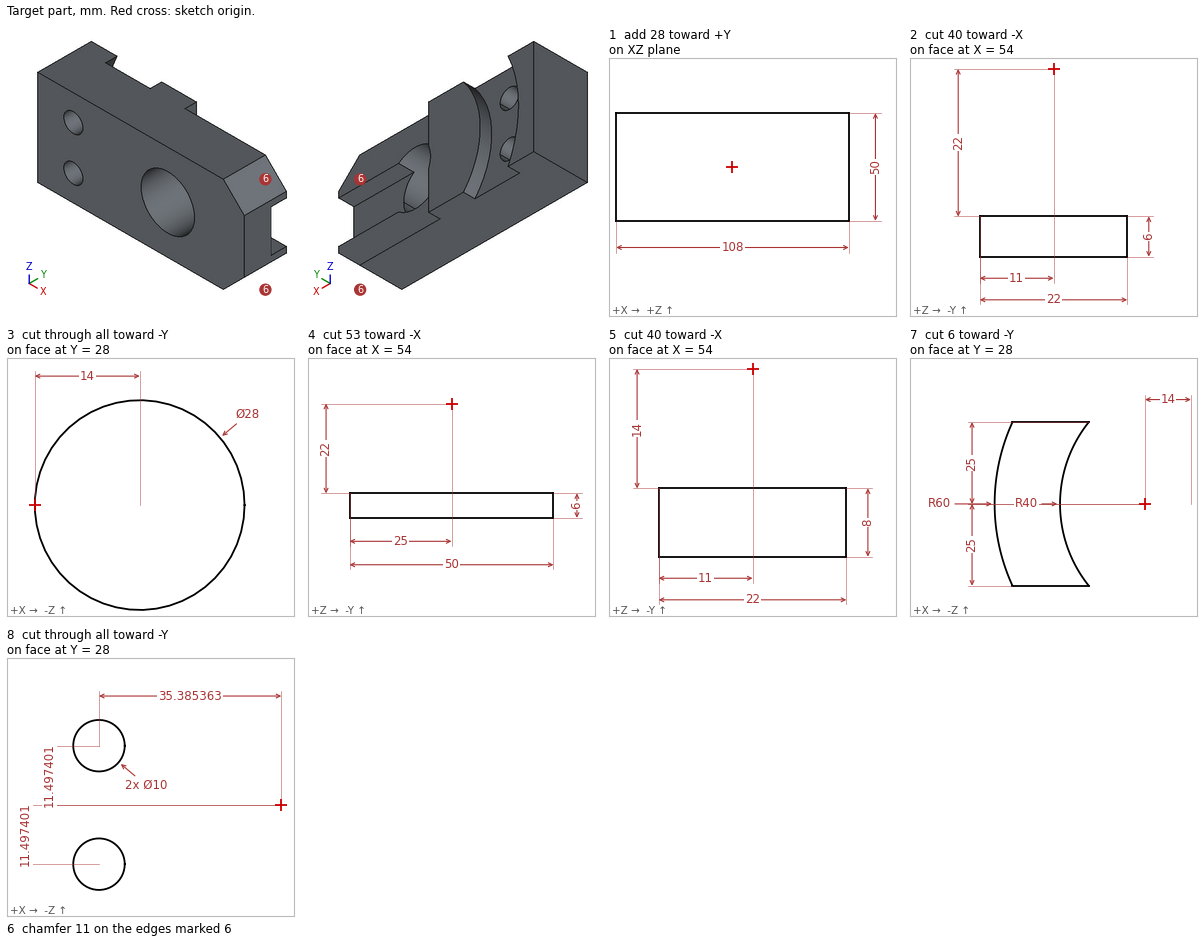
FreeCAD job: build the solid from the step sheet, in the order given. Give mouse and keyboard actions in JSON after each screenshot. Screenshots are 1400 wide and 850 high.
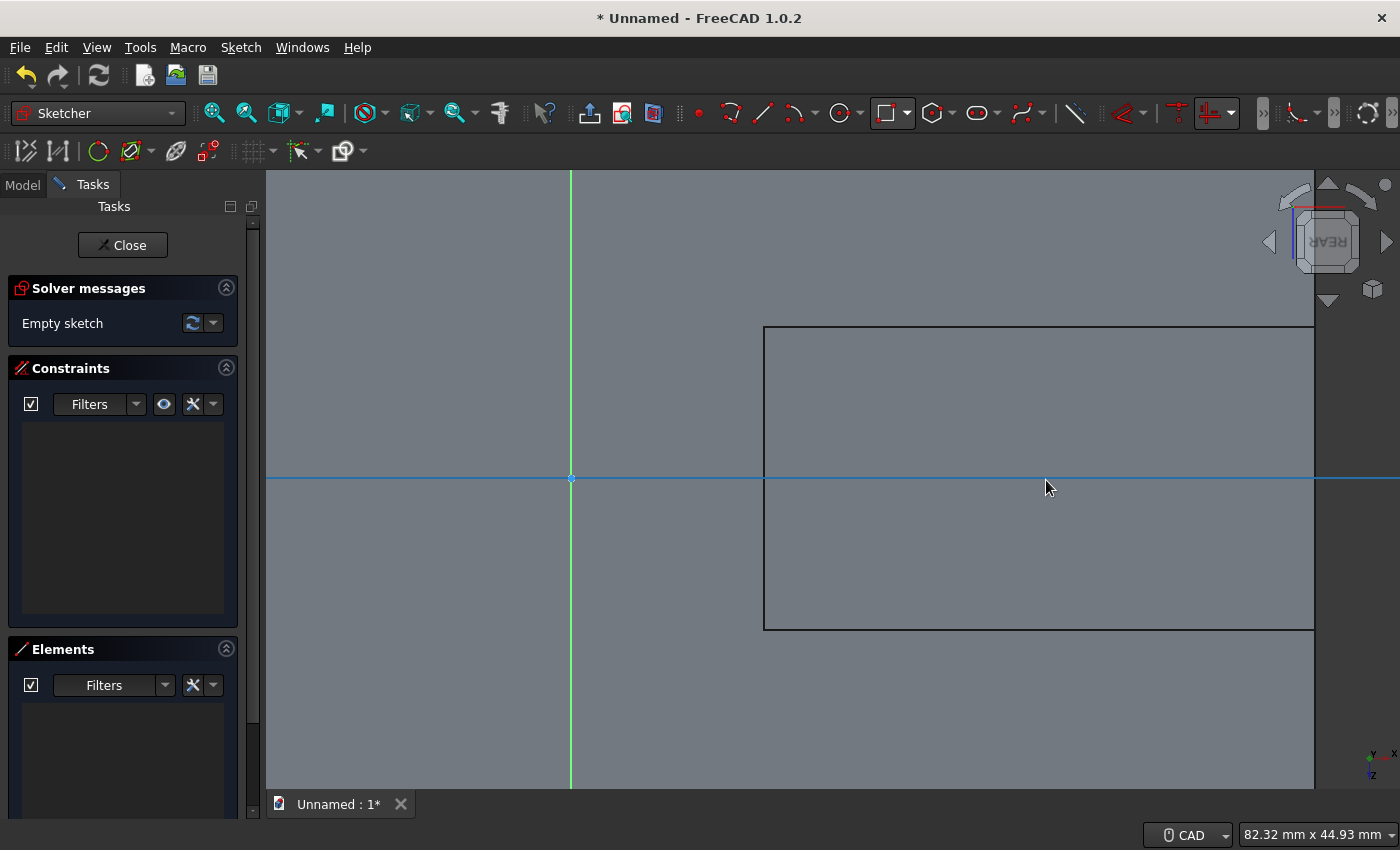
{"action": "key", "text": "g c"}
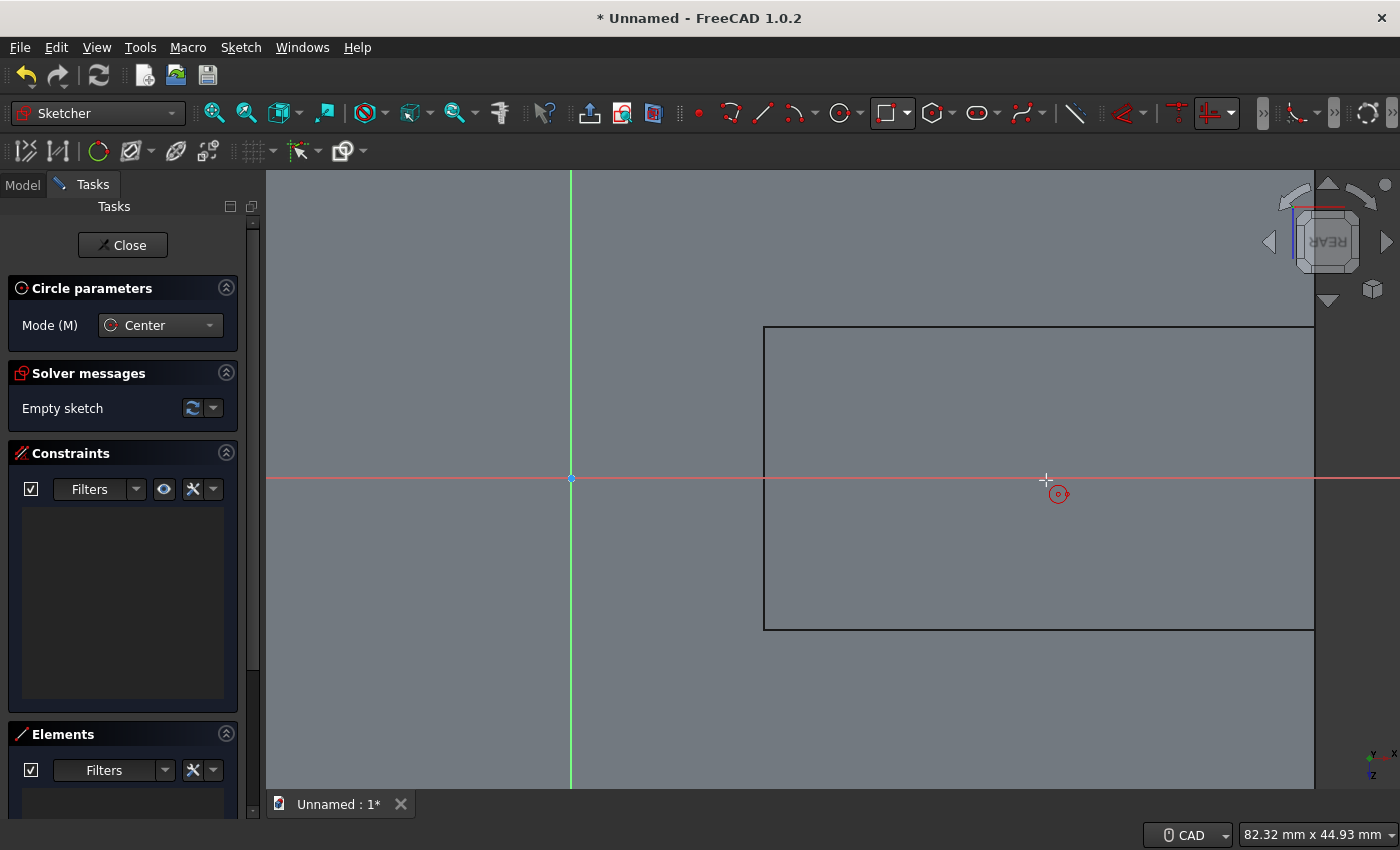
{"action": "left_click", "coordinate": [764, 478]}
{"action": "mouse_move", "coordinate": [900, 342]}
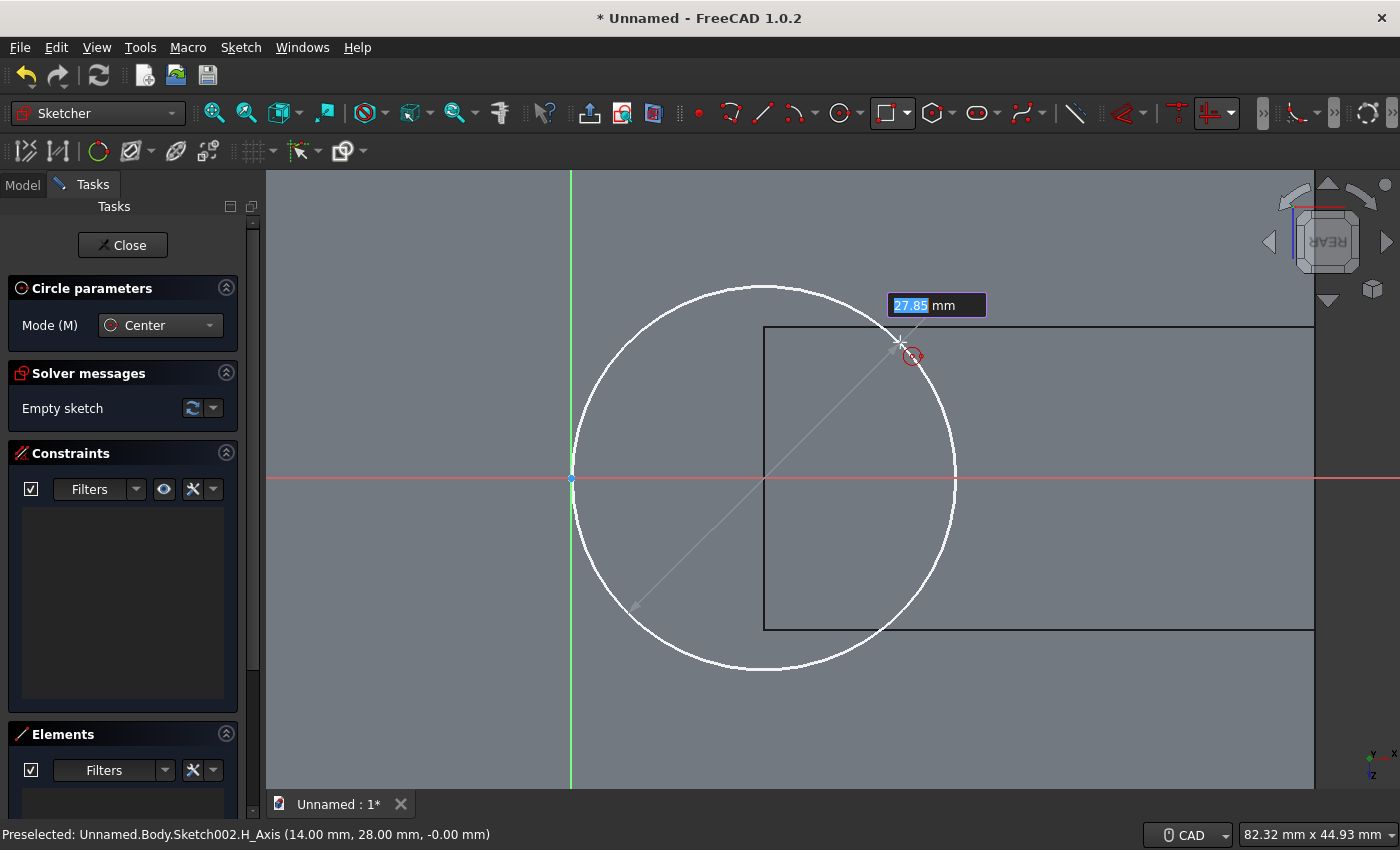
{"action": "type", "text": "28"}
{"action": "key", "text": "Return"}
{"action": "key", "text": "Escape"}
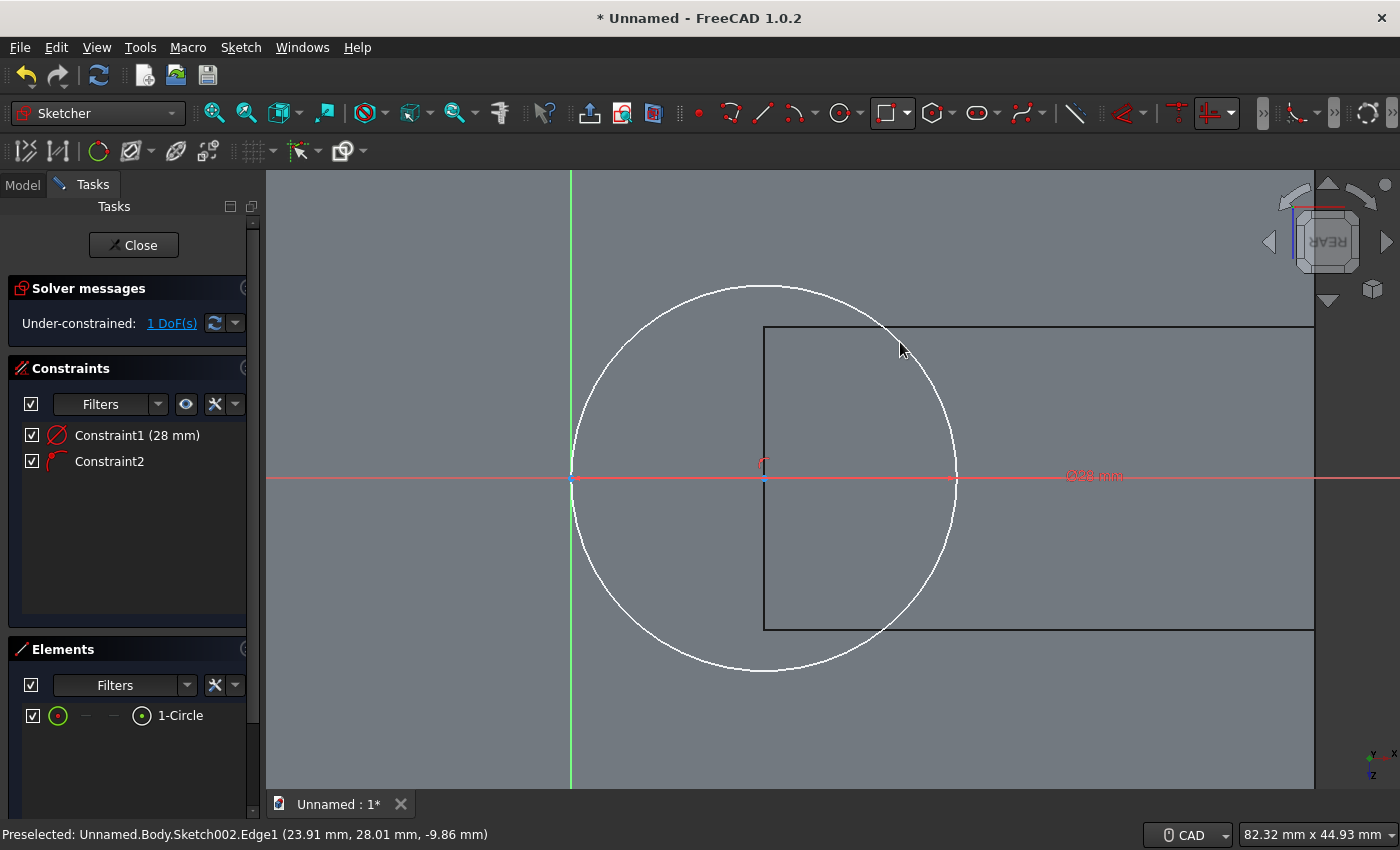
{"action": "key", "text": "d"}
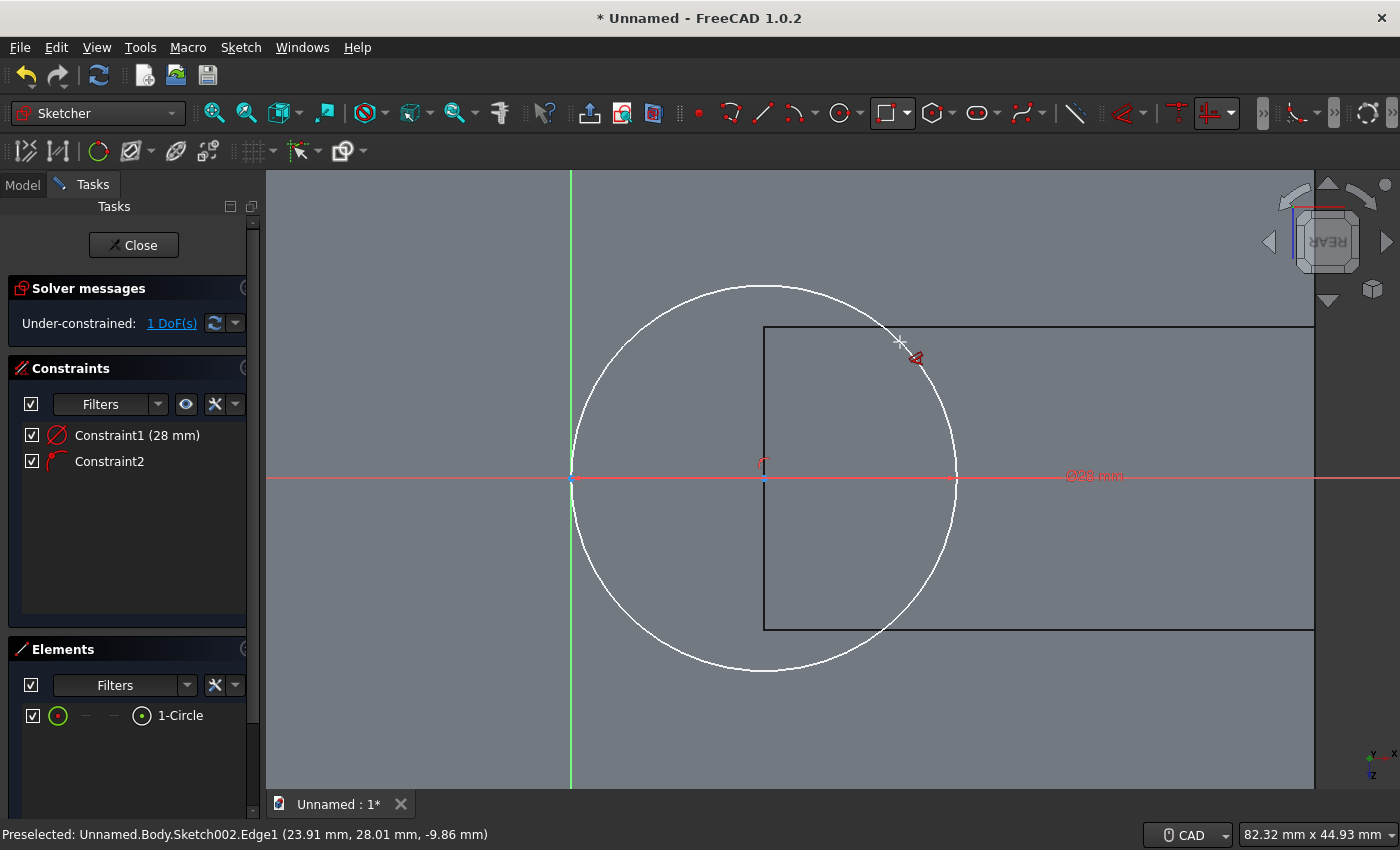
{"action": "left_click", "coordinate": [764, 478]}
{"action": "left_click", "coordinate": [668, 512]}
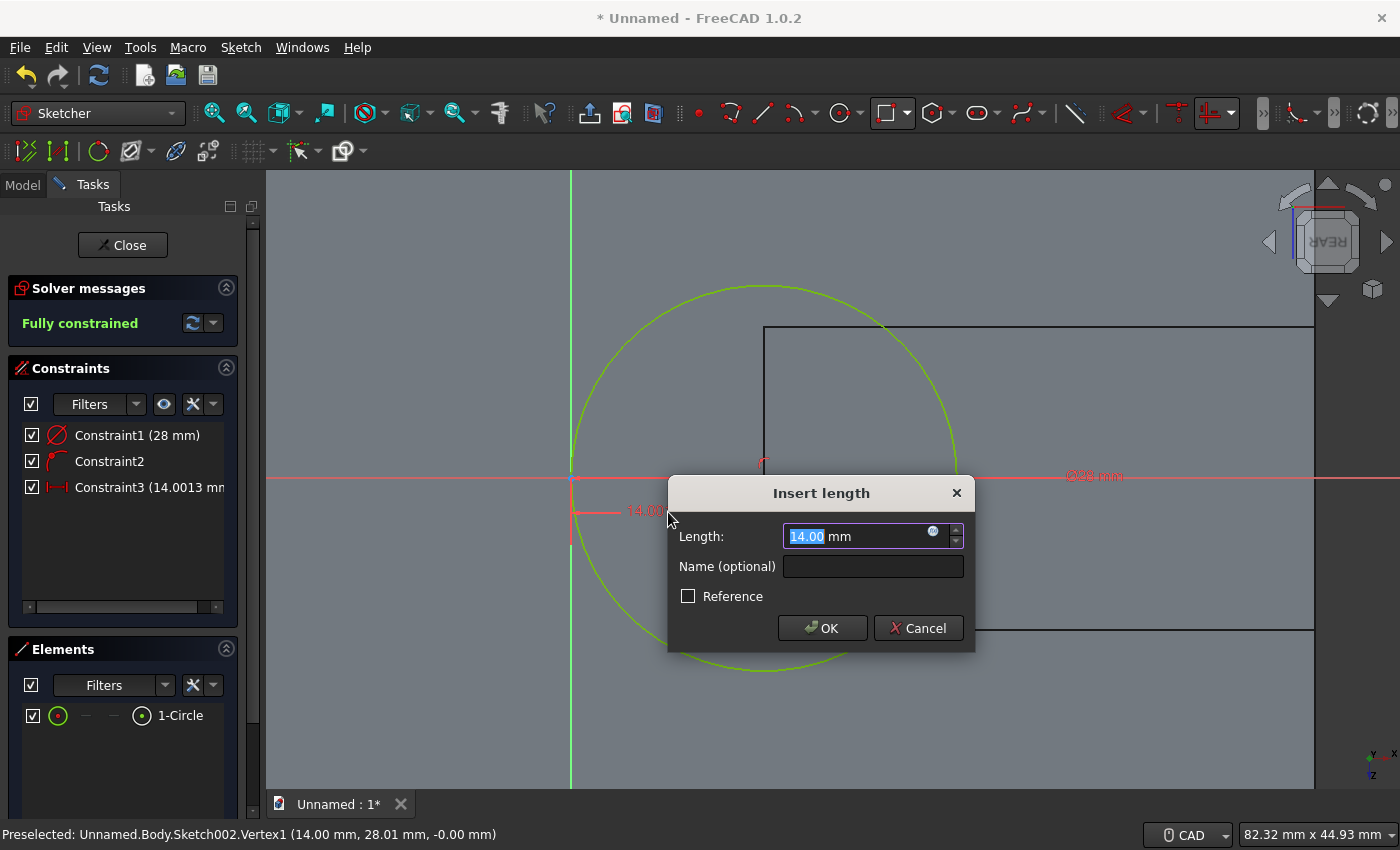
{"action": "type", "text": "14"}
{"action": "key", "text": "Return"}
{"action": "key", "text": "Escape"}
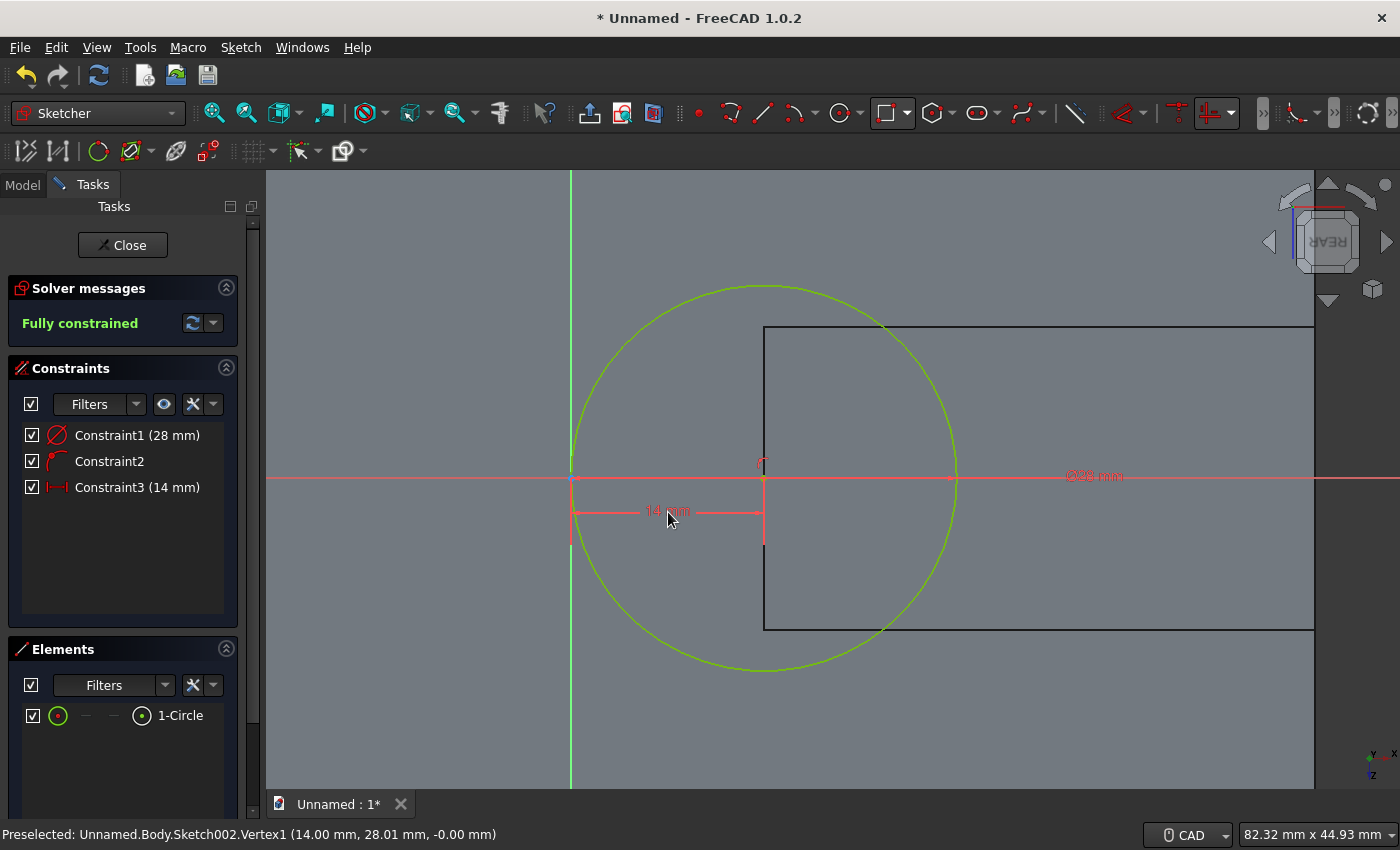
{"action": "left_click", "coordinate": [123, 245]}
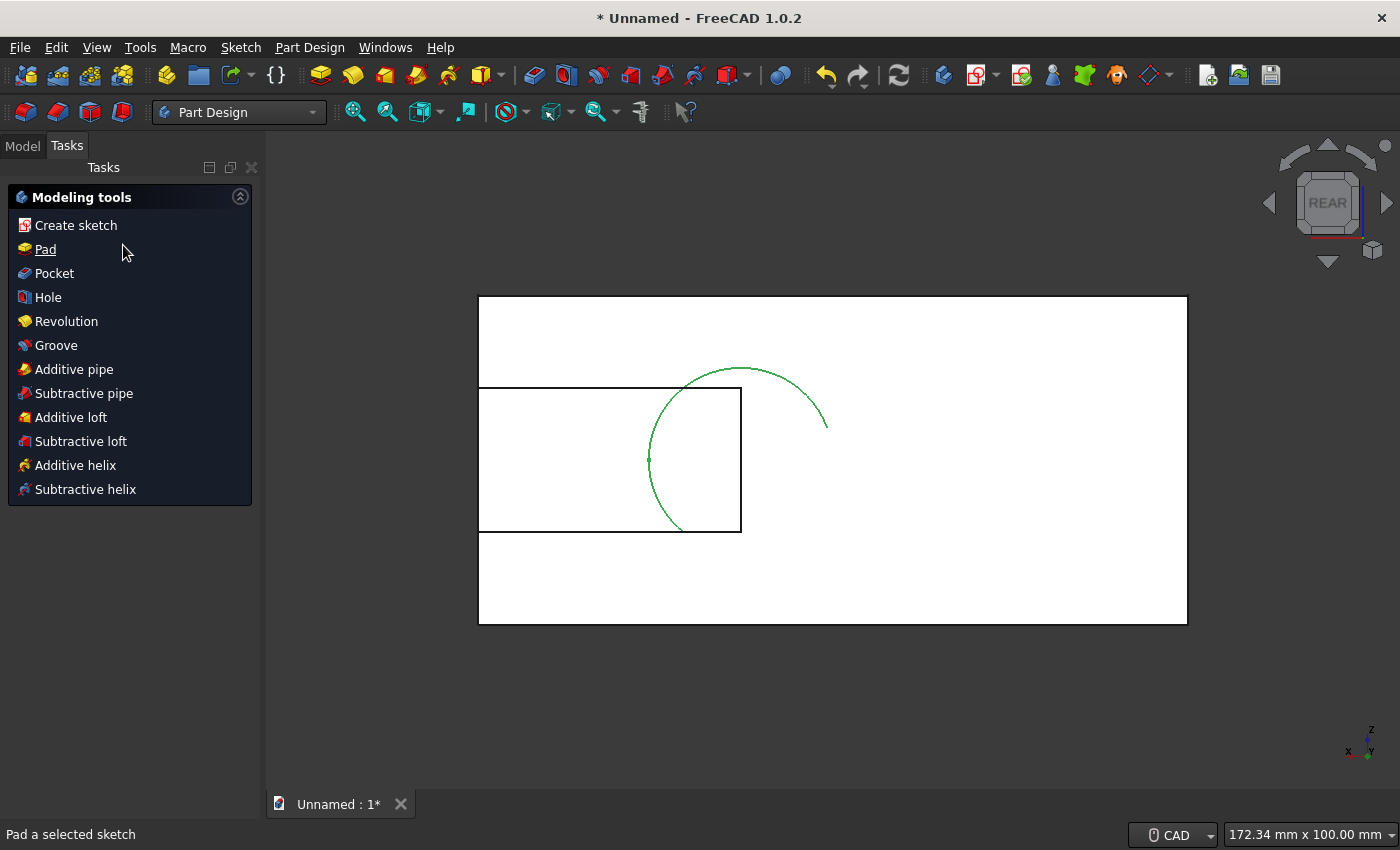
{"action": "left_click", "coordinate": [536, 76]}